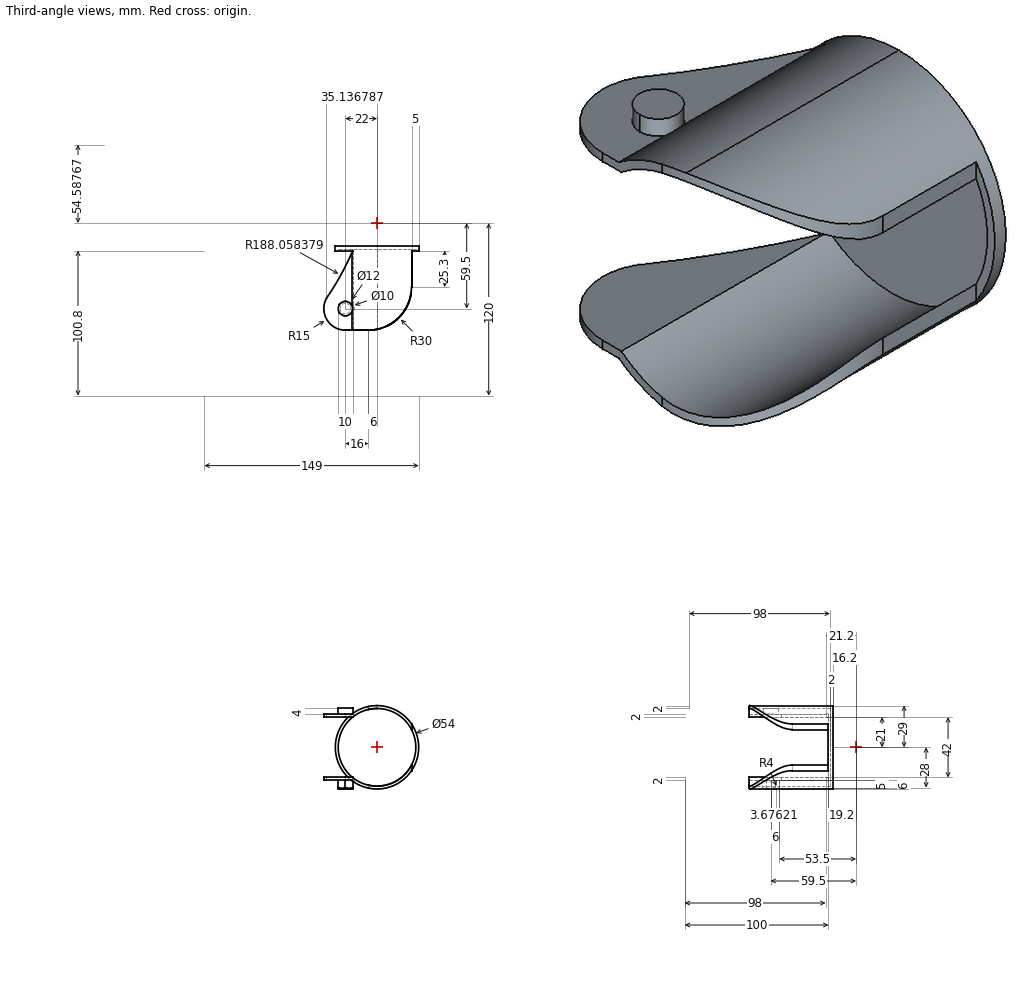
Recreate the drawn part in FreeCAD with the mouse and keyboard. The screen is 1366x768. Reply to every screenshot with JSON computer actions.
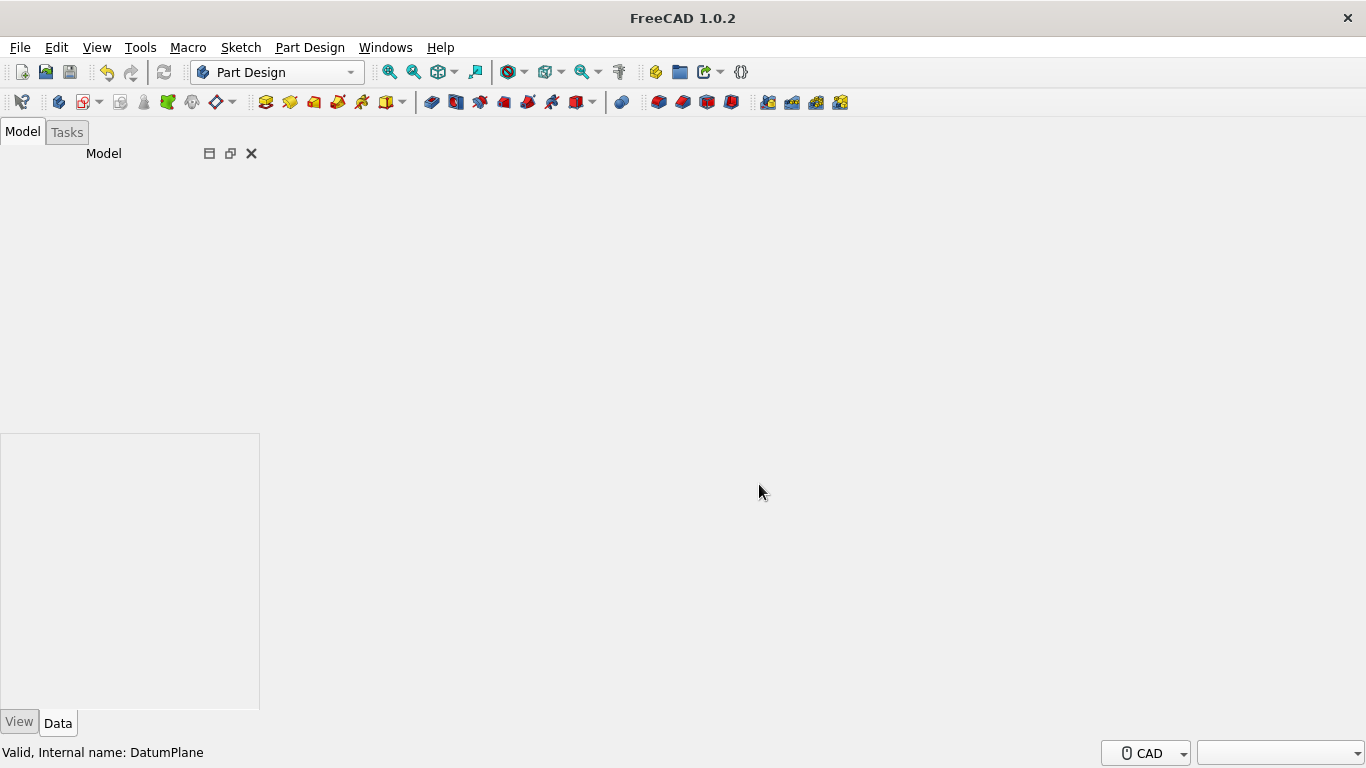
{"action": "left_click", "coordinate": [22, 72]}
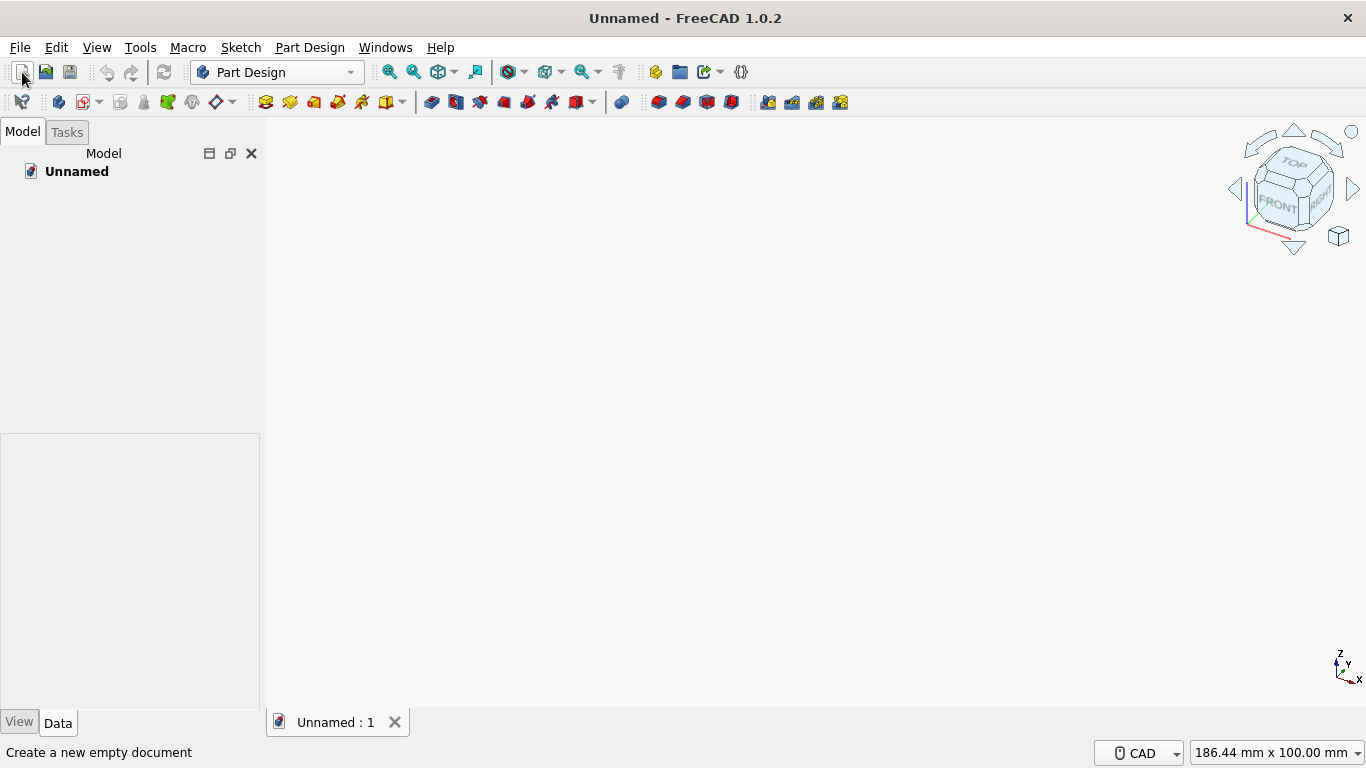
{"action": "left_click", "coordinate": [84, 102]}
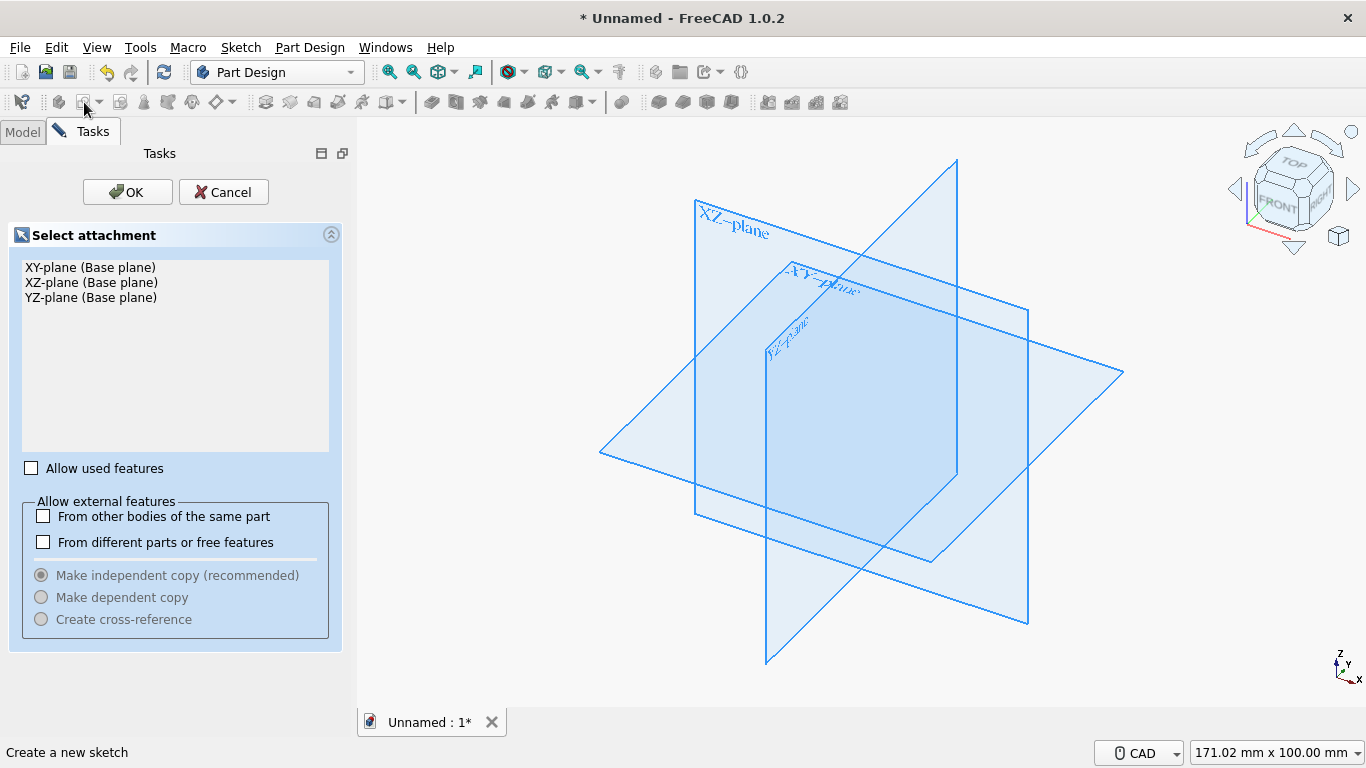
{"action": "left_click", "coordinate": [82, 298]}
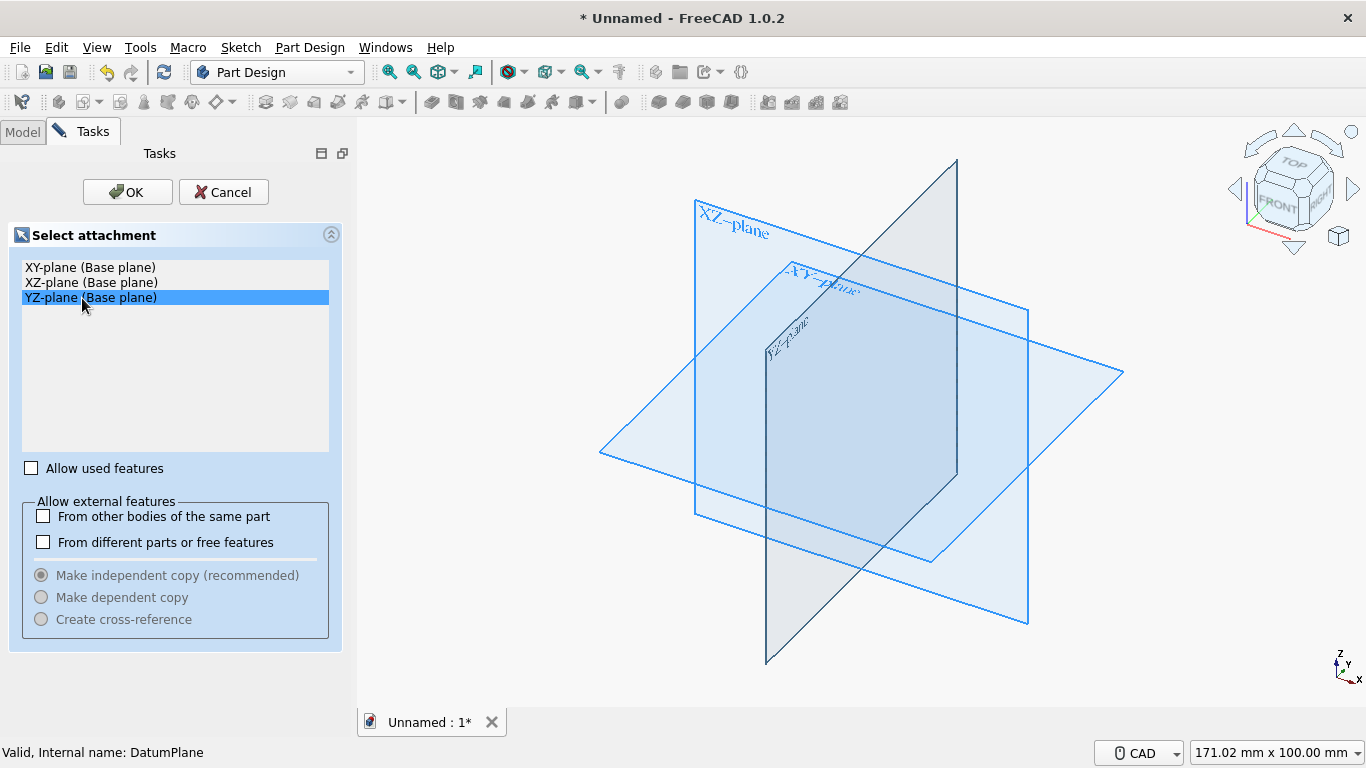
{"action": "left_click", "coordinate": [128, 192]}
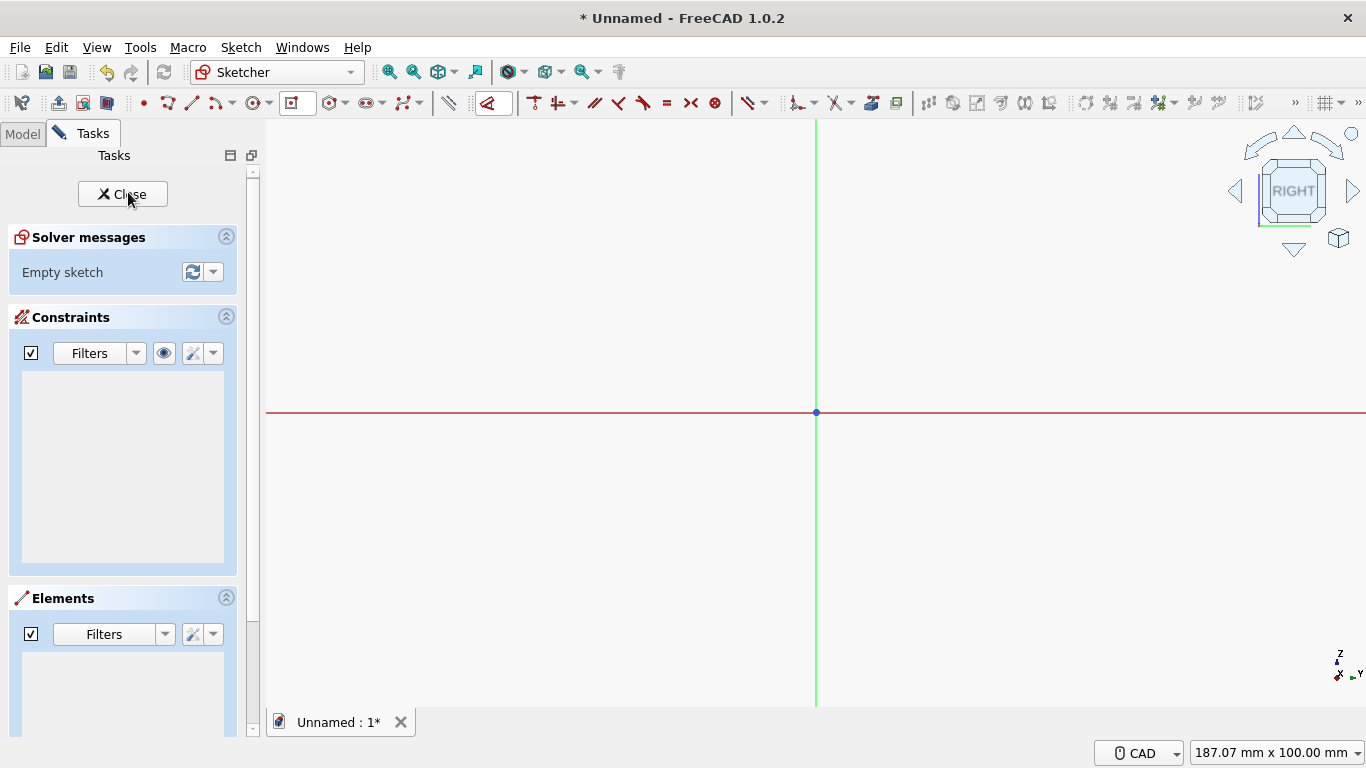
{"action": "scroll", "coordinate": [1201, 679], "scroll_direction": "down", "scroll_amount": 1}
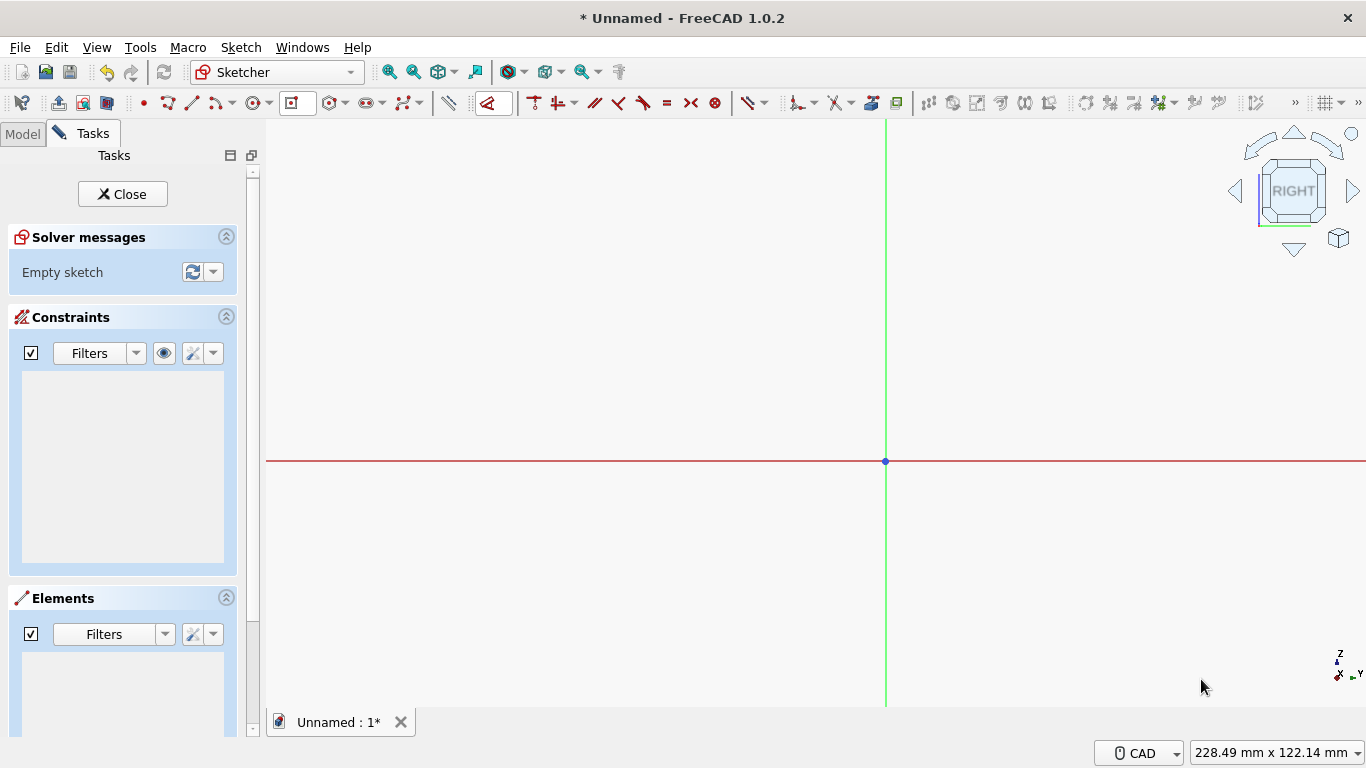
{"action": "left_click", "coordinate": [168, 104]}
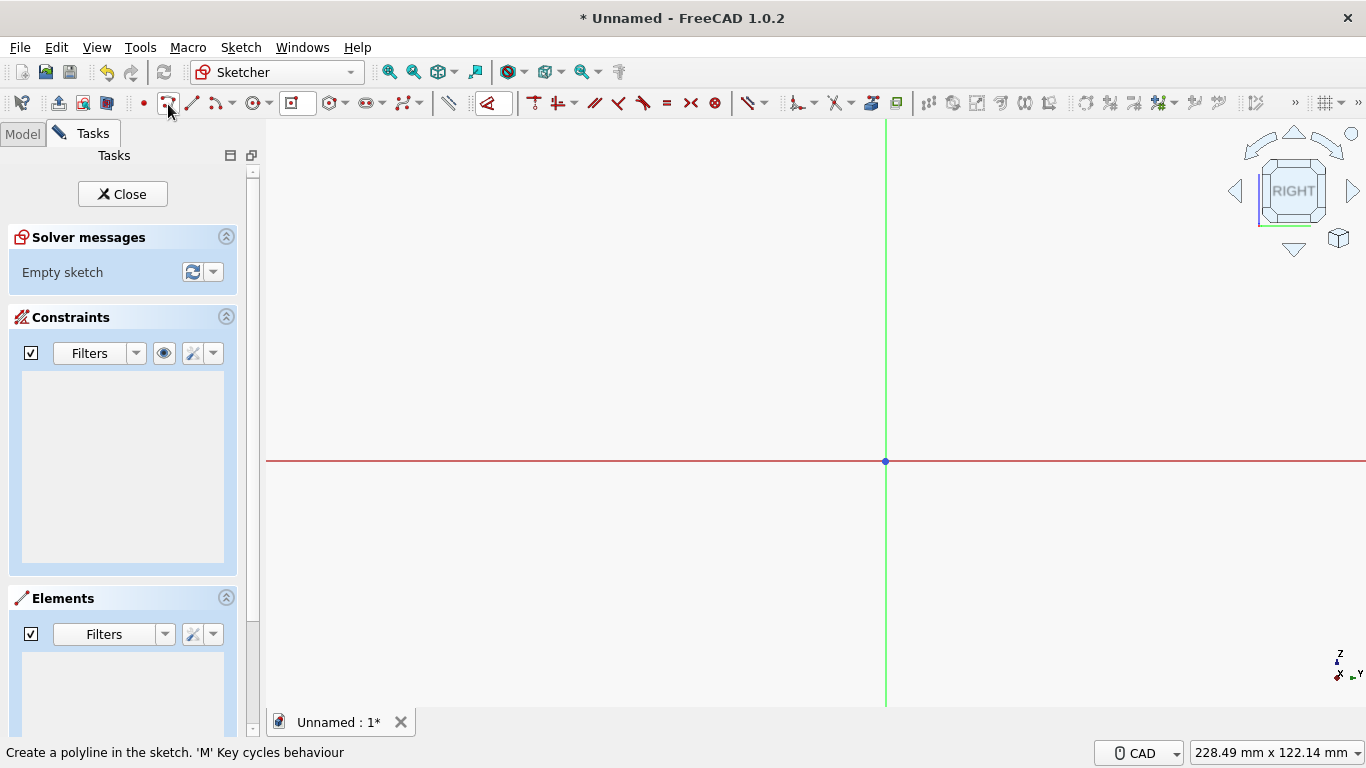
{"action": "left_click", "coordinate": [808, 461]}
{"action": "left_click", "coordinate": [808, 322]}
{"action": "left_click", "coordinate": [327, 322]}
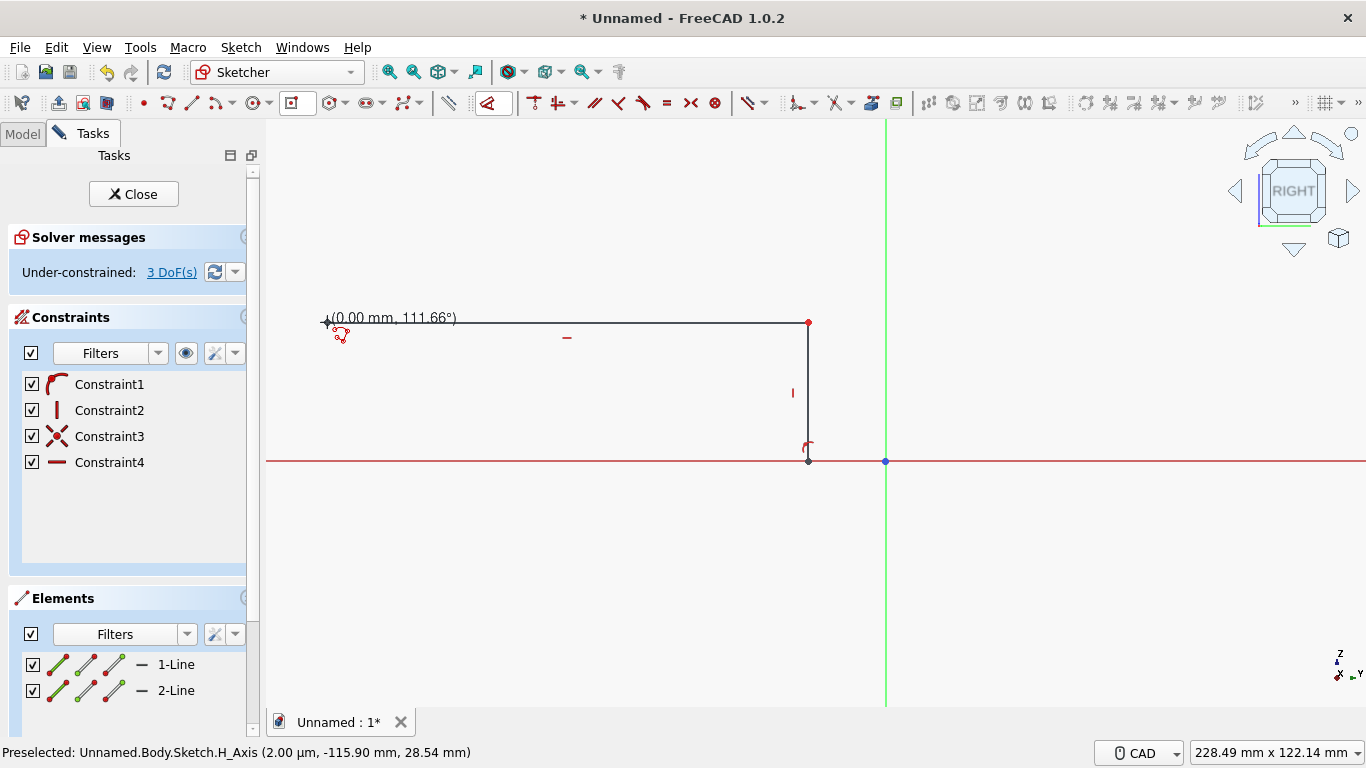
{"action": "scroll", "coordinate": [327, 331], "scroll_direction": "up", "scroll_amount": 3}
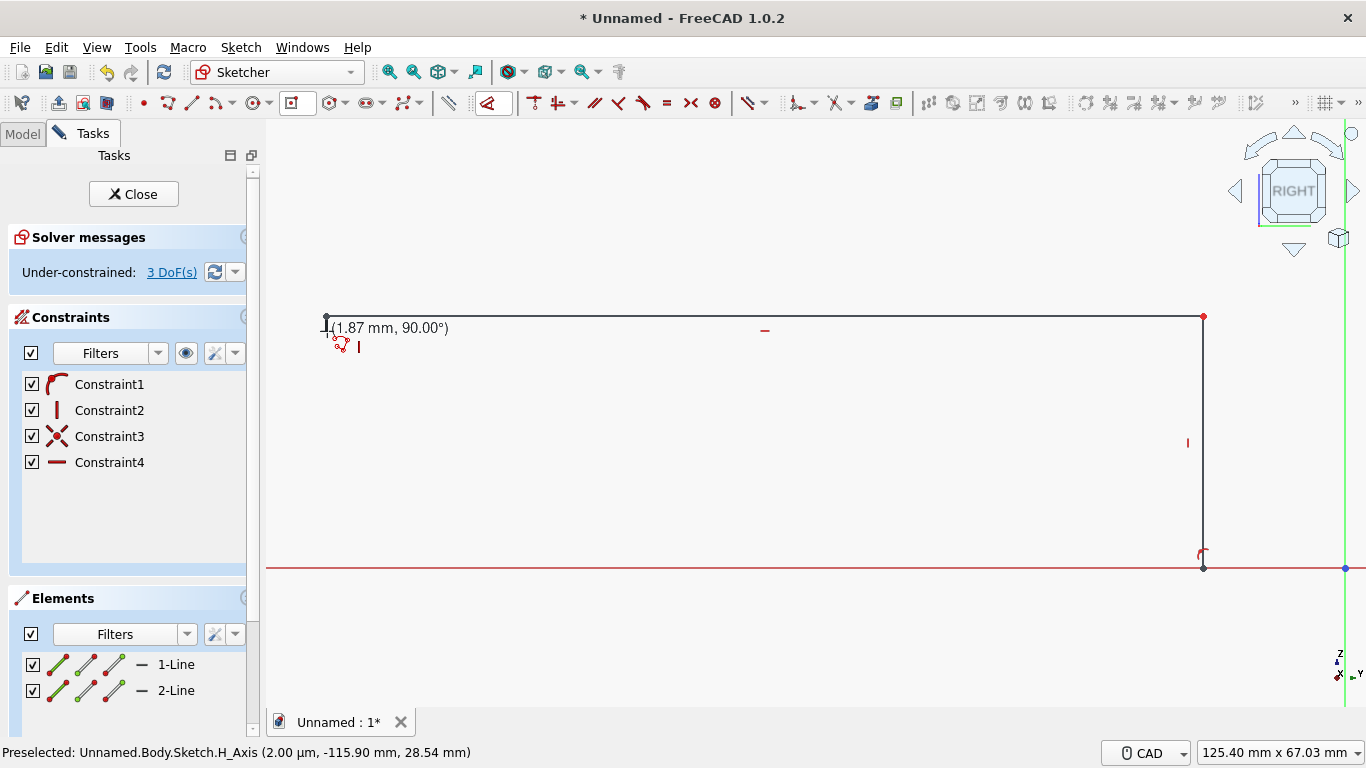
{"action": "left_click", "coordinate": [327, 331]}
{"action": "left_click", "coordinate": [1186, 331]}
{"action": "left_click", "coordinate": [1186, 559]}